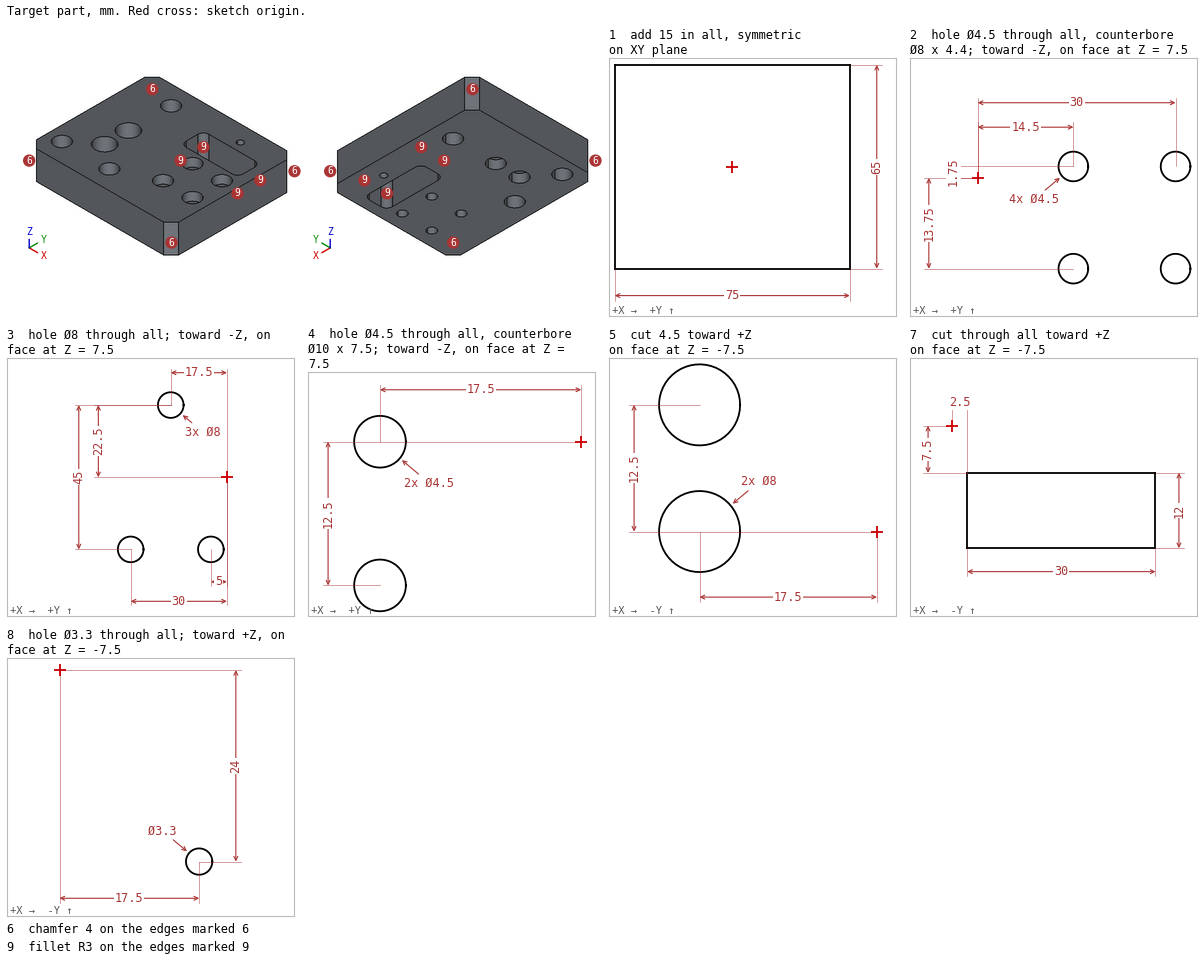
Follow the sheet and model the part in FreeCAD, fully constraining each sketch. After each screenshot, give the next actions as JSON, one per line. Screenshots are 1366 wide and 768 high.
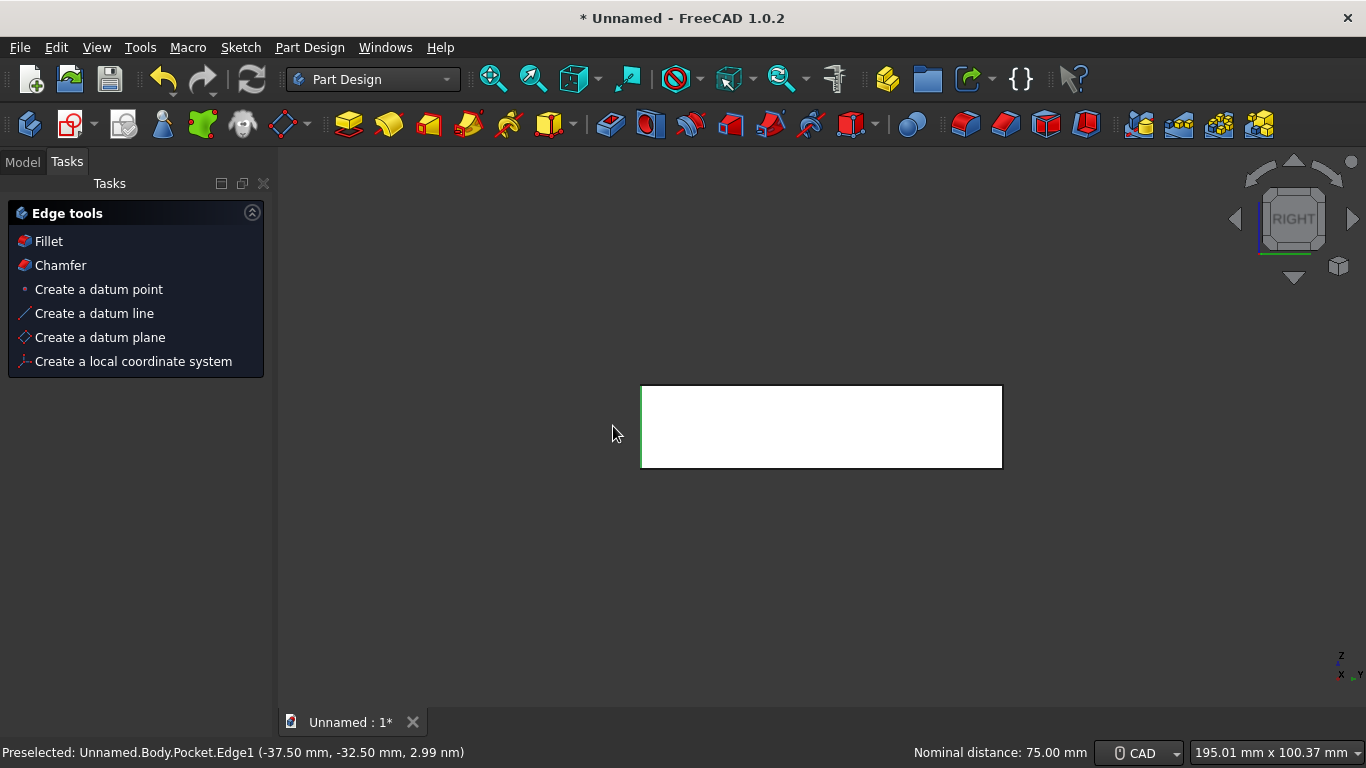
{"action": "key", "text": "v f"}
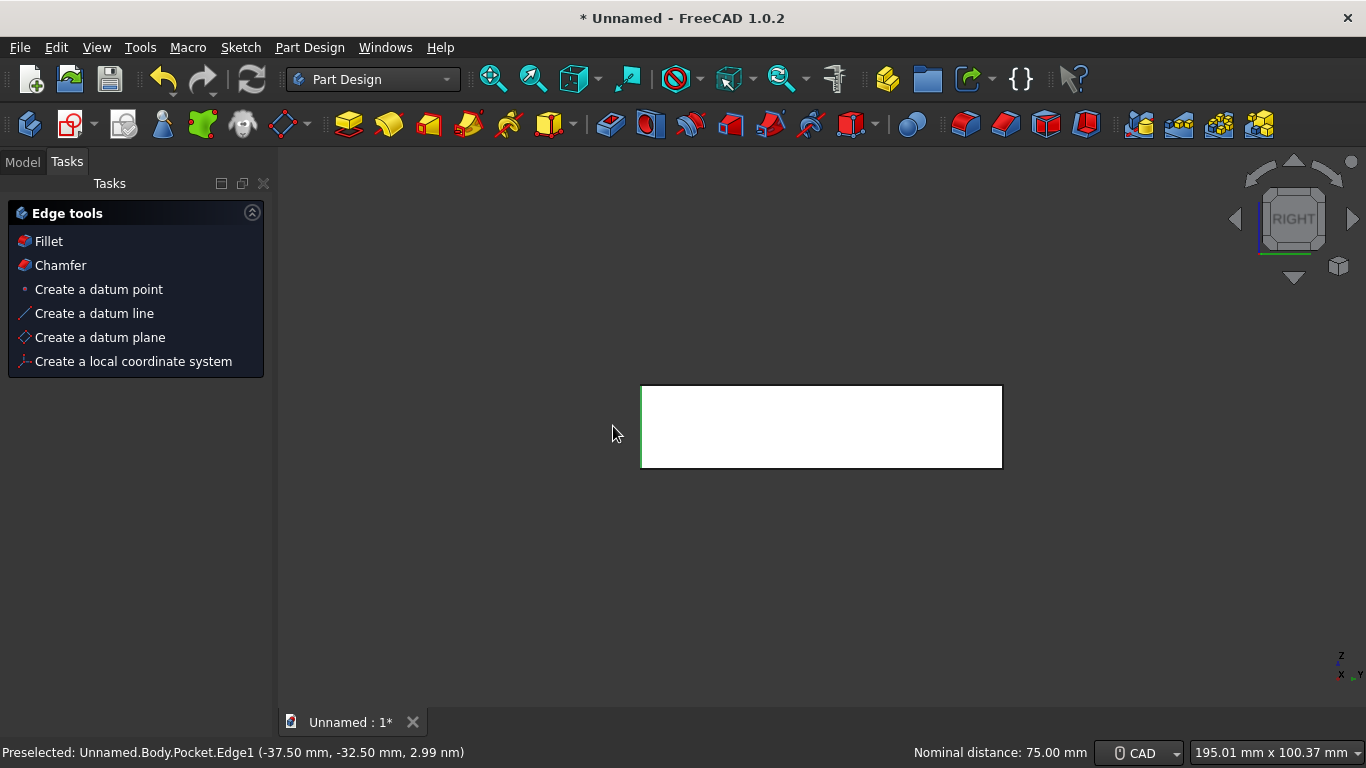
{"action": "left_click", "coordinate": [1003, 426], "text": "ctrl"}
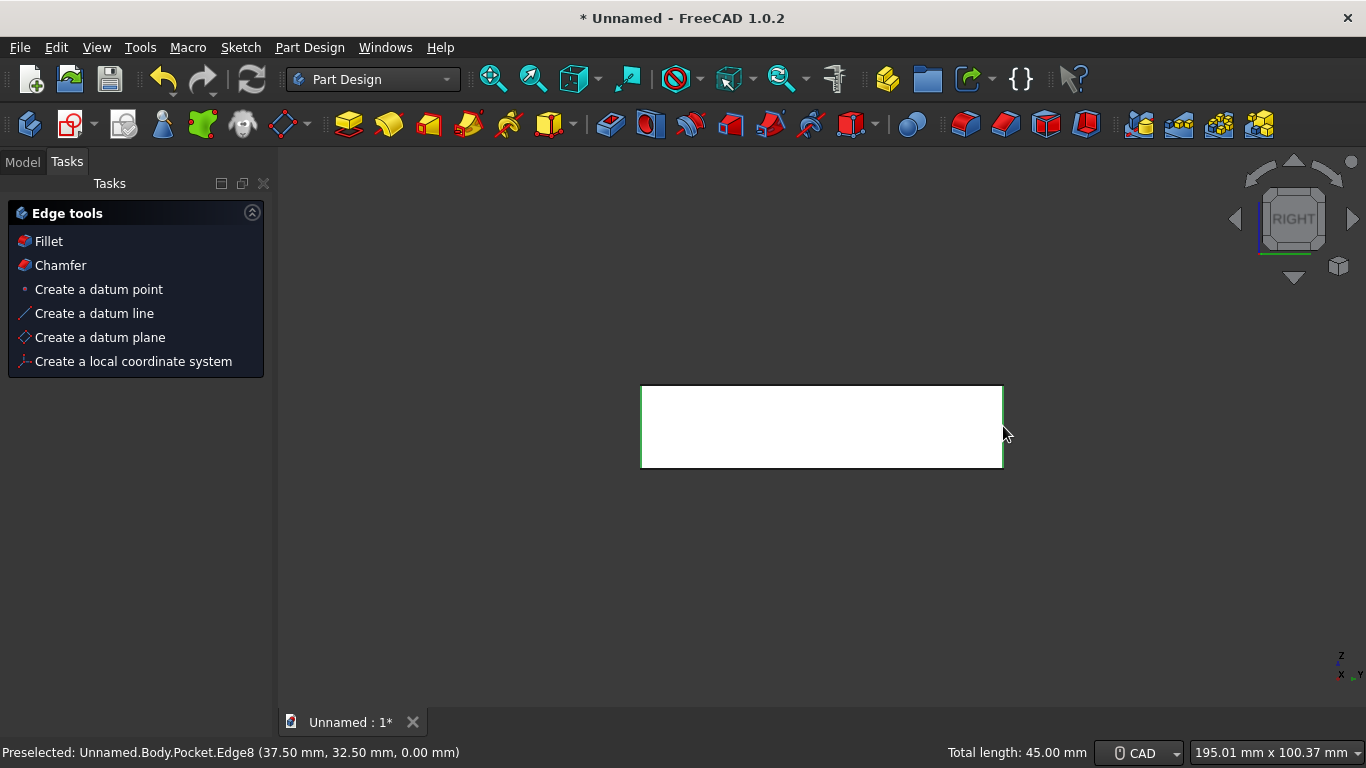
{"action": "key", "text": "5"}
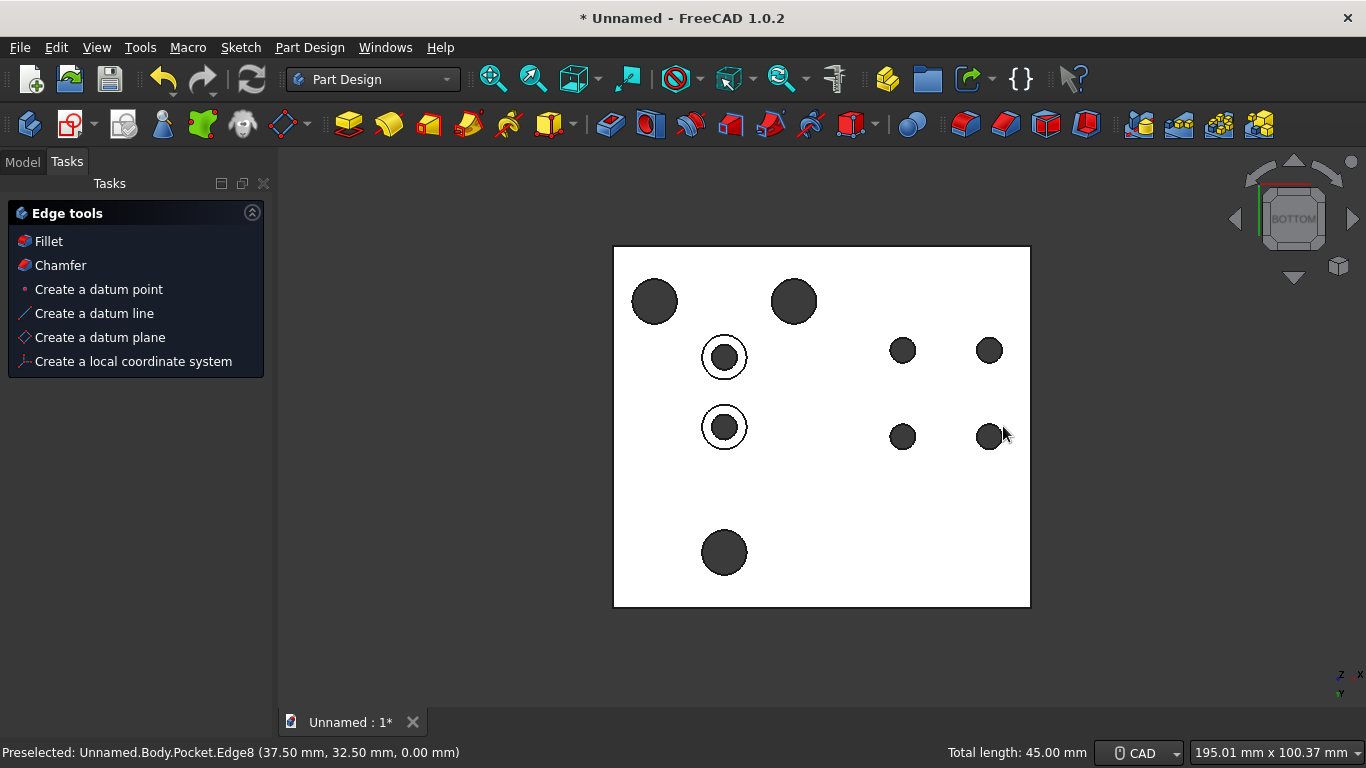
{"action": "key", "text": "4"}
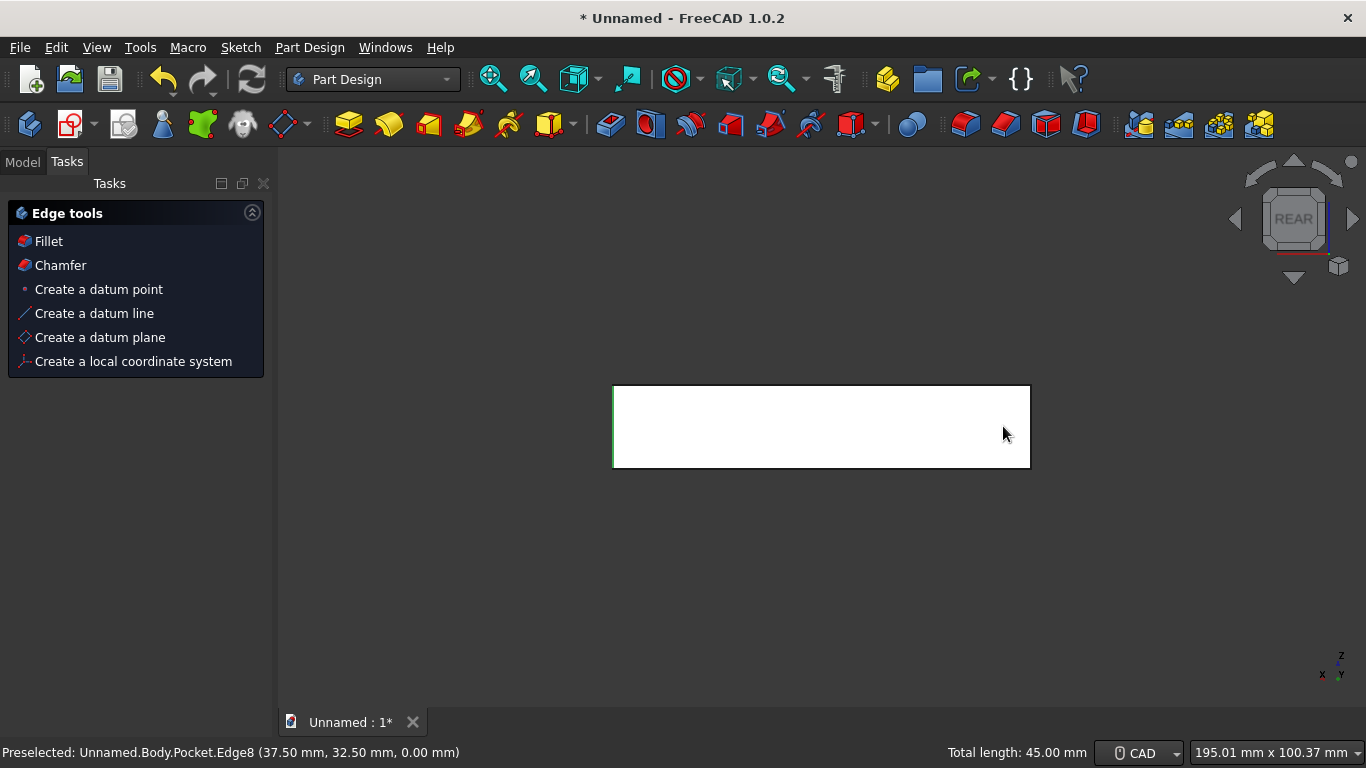
{"action": "key", "text": "v f"}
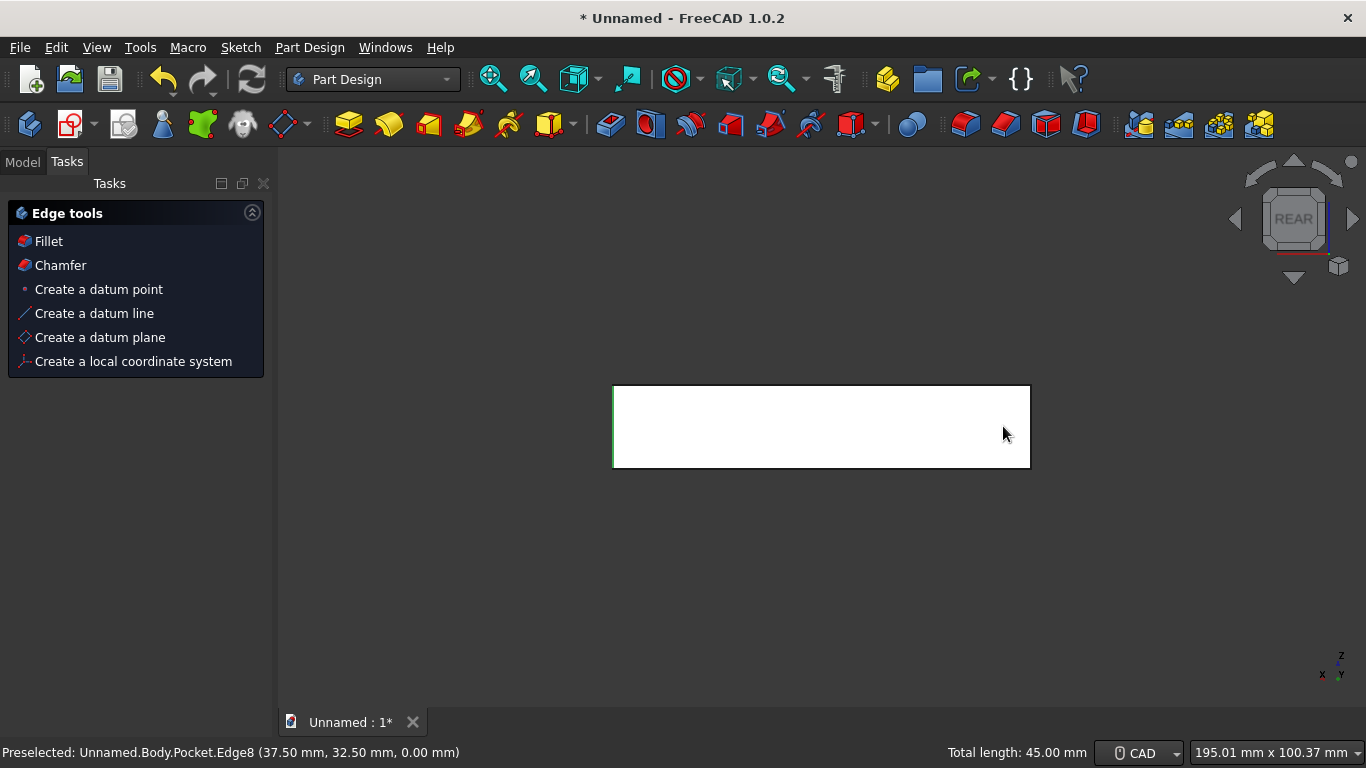
{"action": "left_click", "coordinate": [1031, 426], "text": "ctrl"}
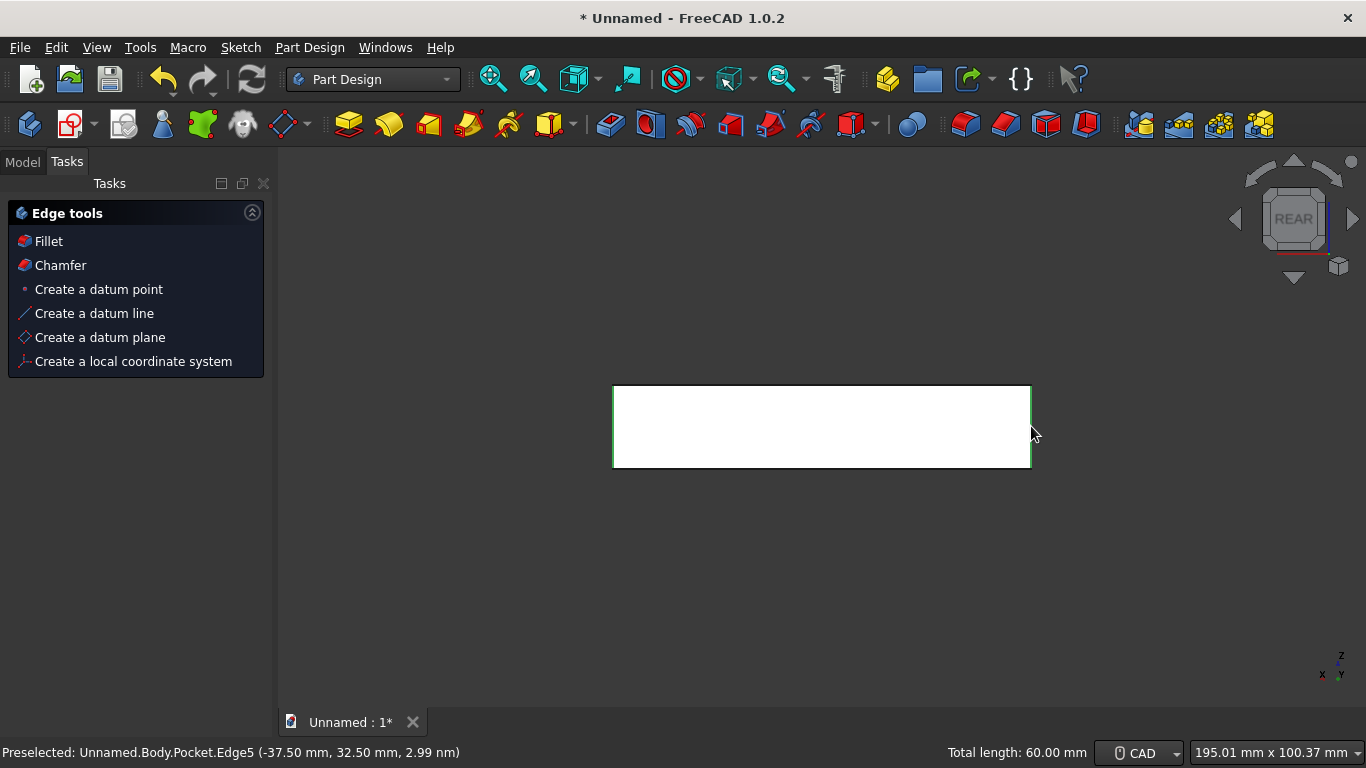
{"action": "left_click", "coordinate": [1006, 124]}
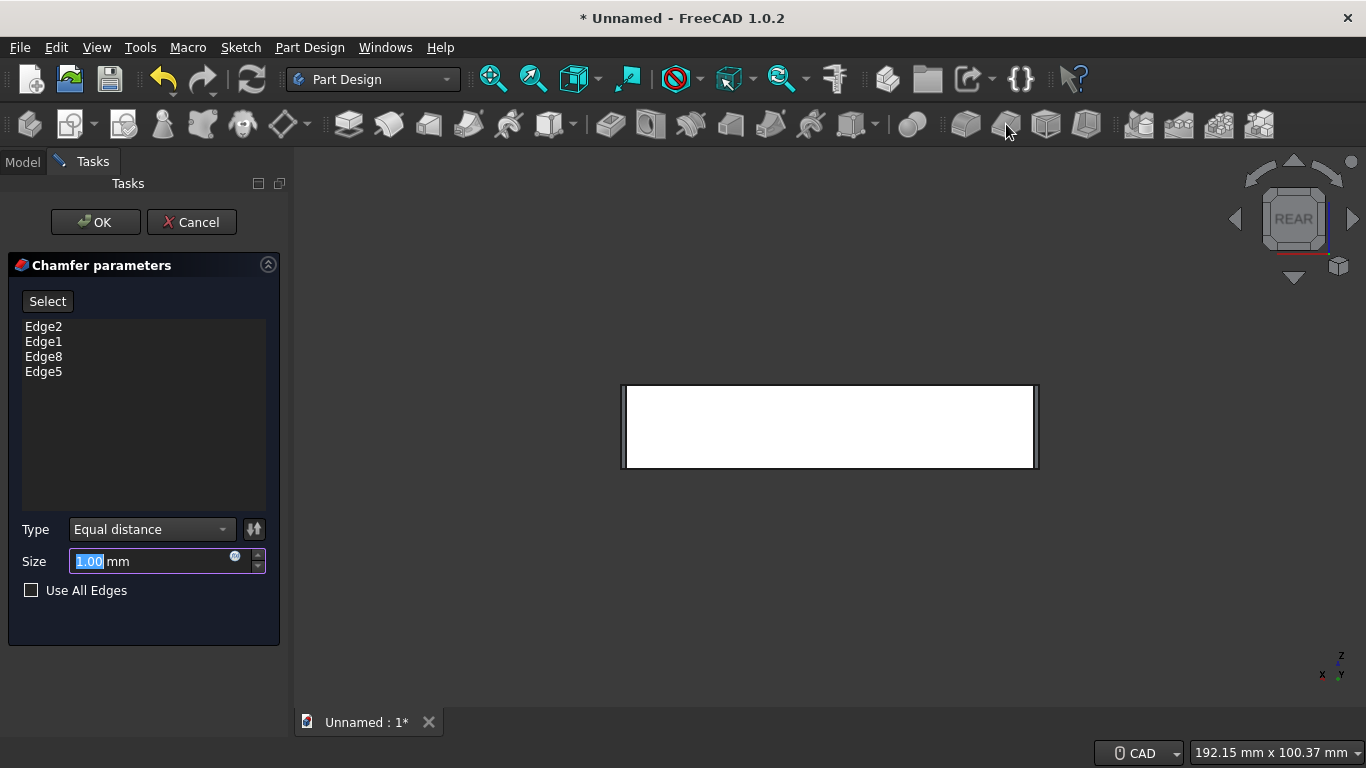
{"action": "type", "text": "4"}
{"action": "key", "text": "Tab"}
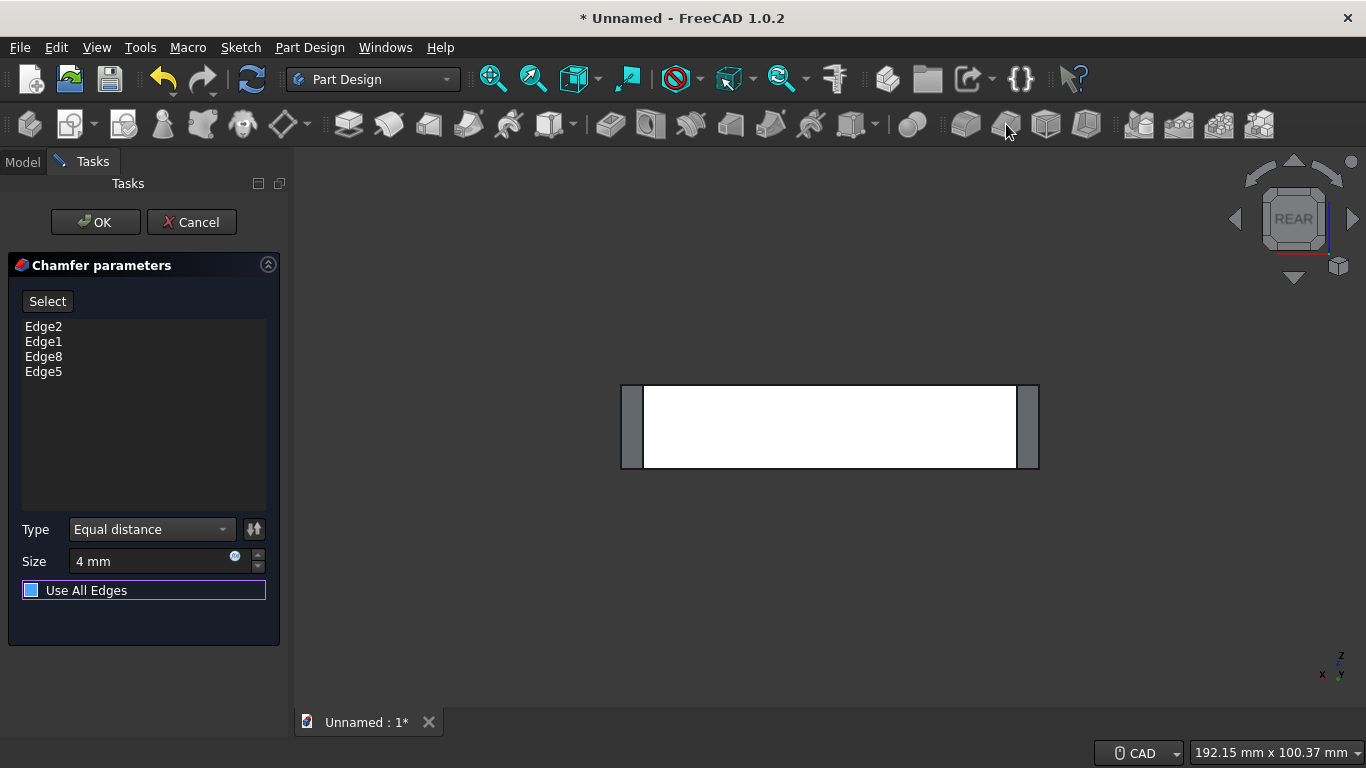
{"action": "left_click", "coordinate": [96, 222]}